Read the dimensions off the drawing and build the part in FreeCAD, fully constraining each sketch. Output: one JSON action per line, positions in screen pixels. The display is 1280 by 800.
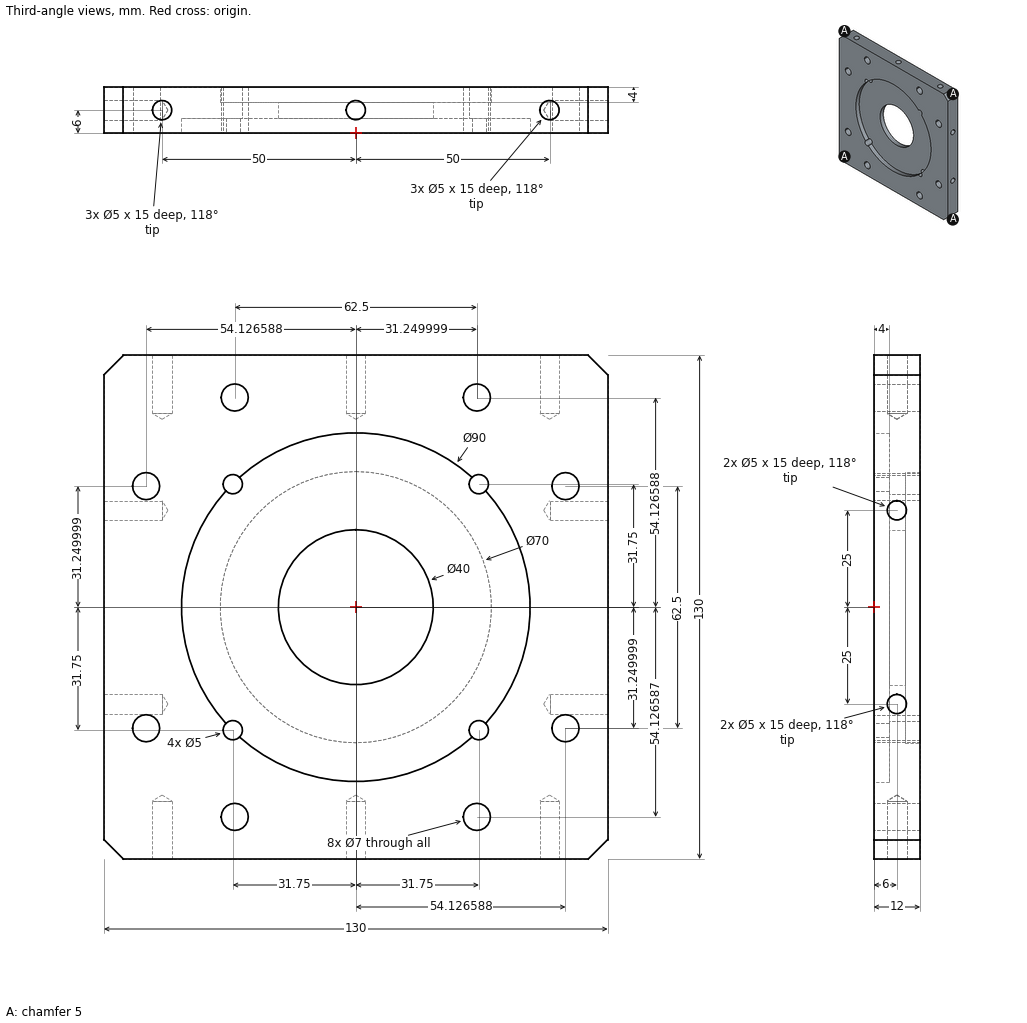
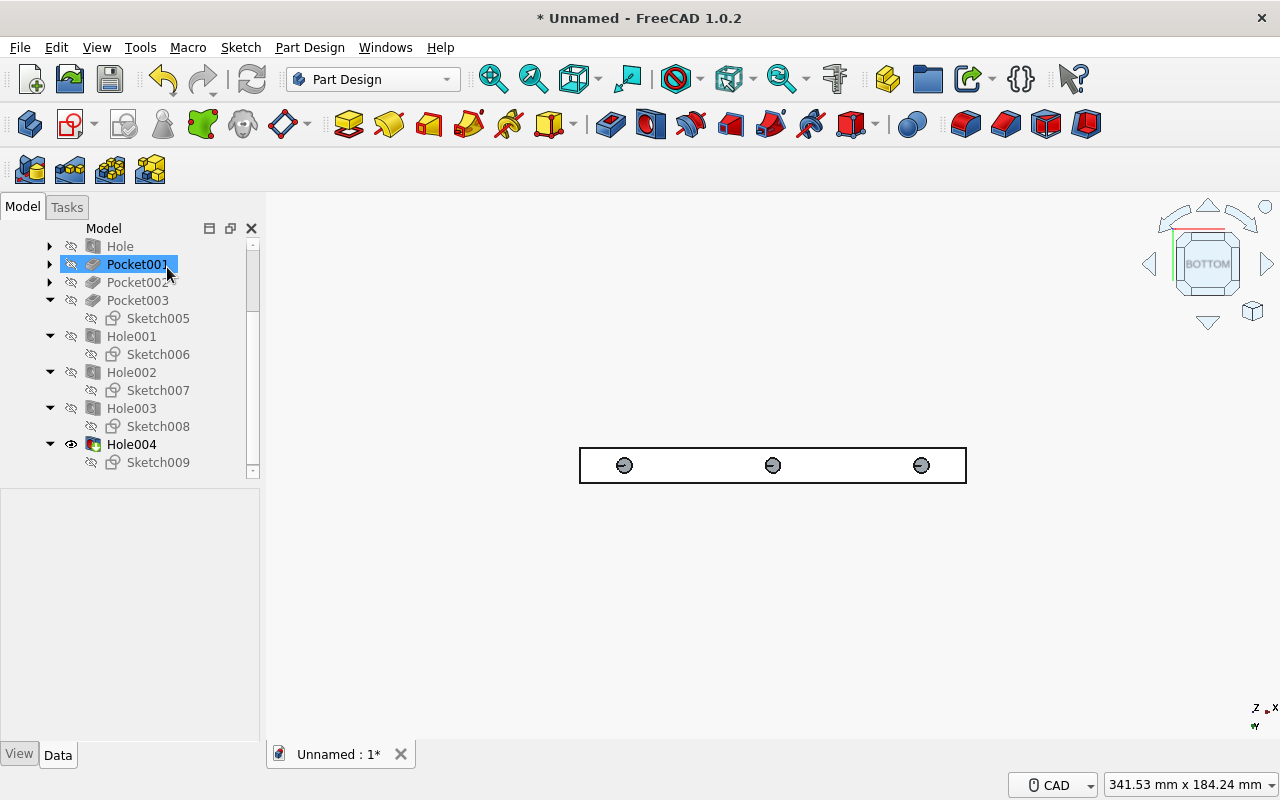
{"action": "left_click", "coordinate": [580, 464]}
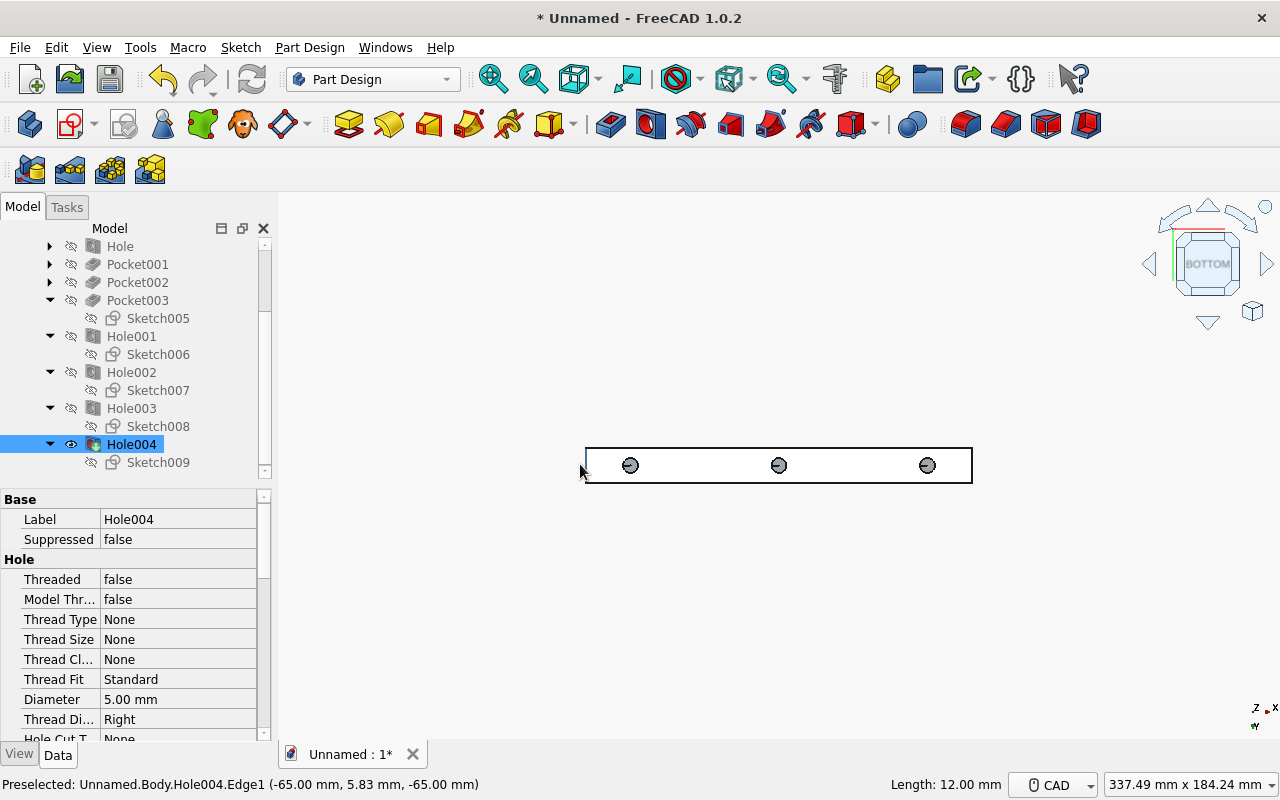
{"action": "left_click", "coordinate": [972, 464], "text": "ctrl"}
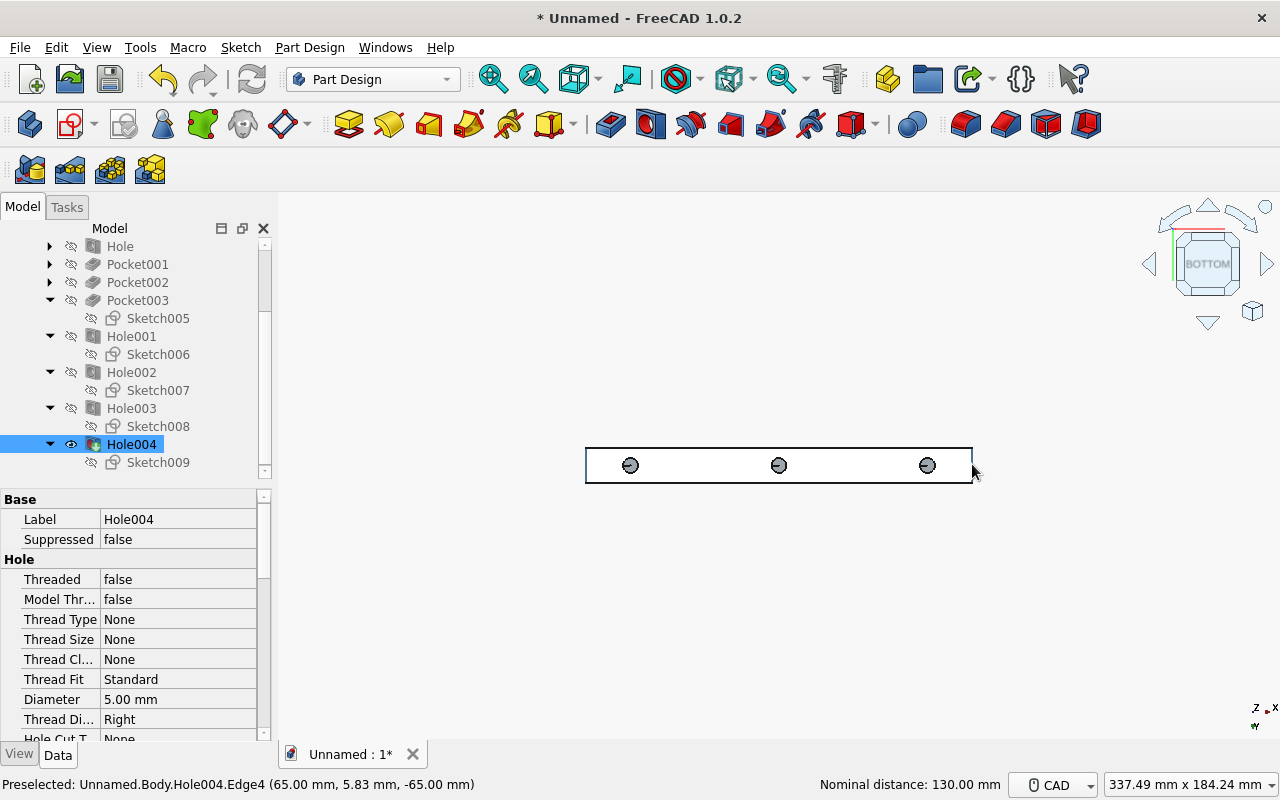
{"action": "key", "text": "0"}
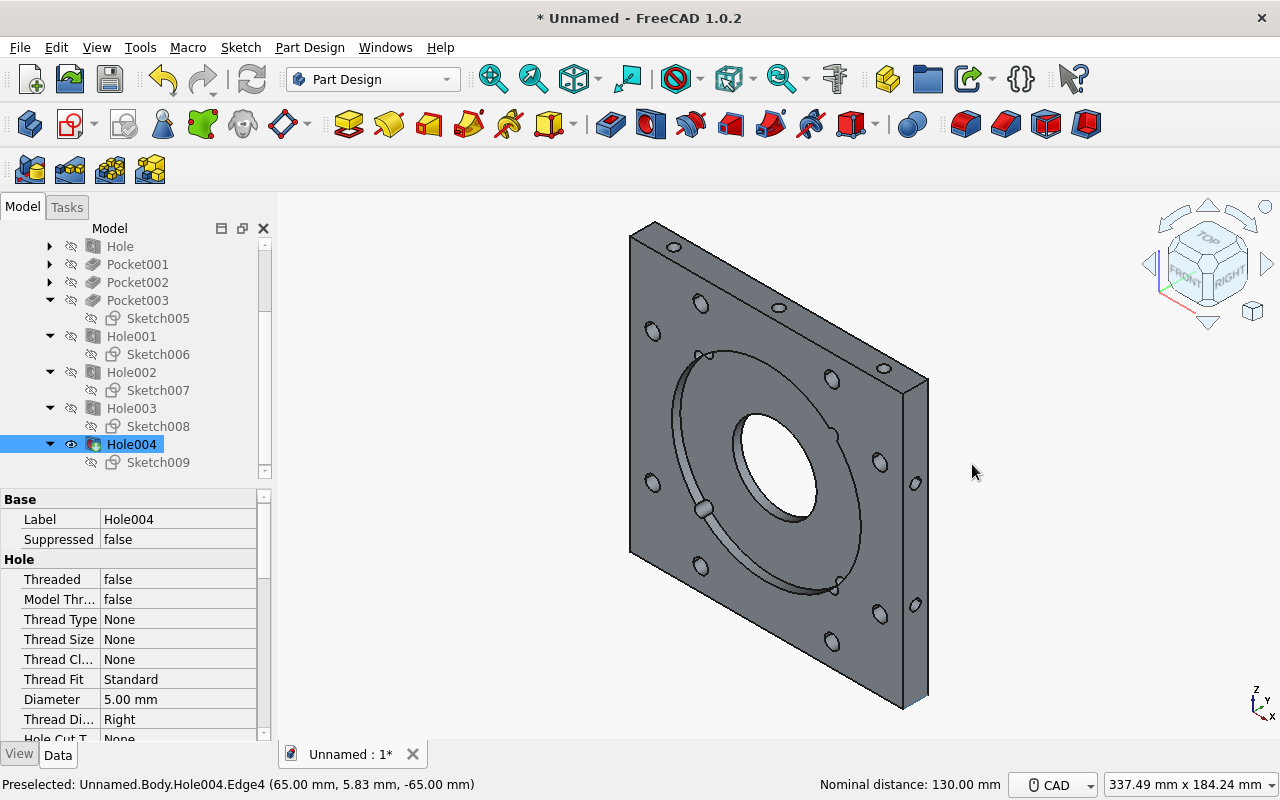
{"action": "left_click", "coordinate": [915, 386], "text": "ctrl"}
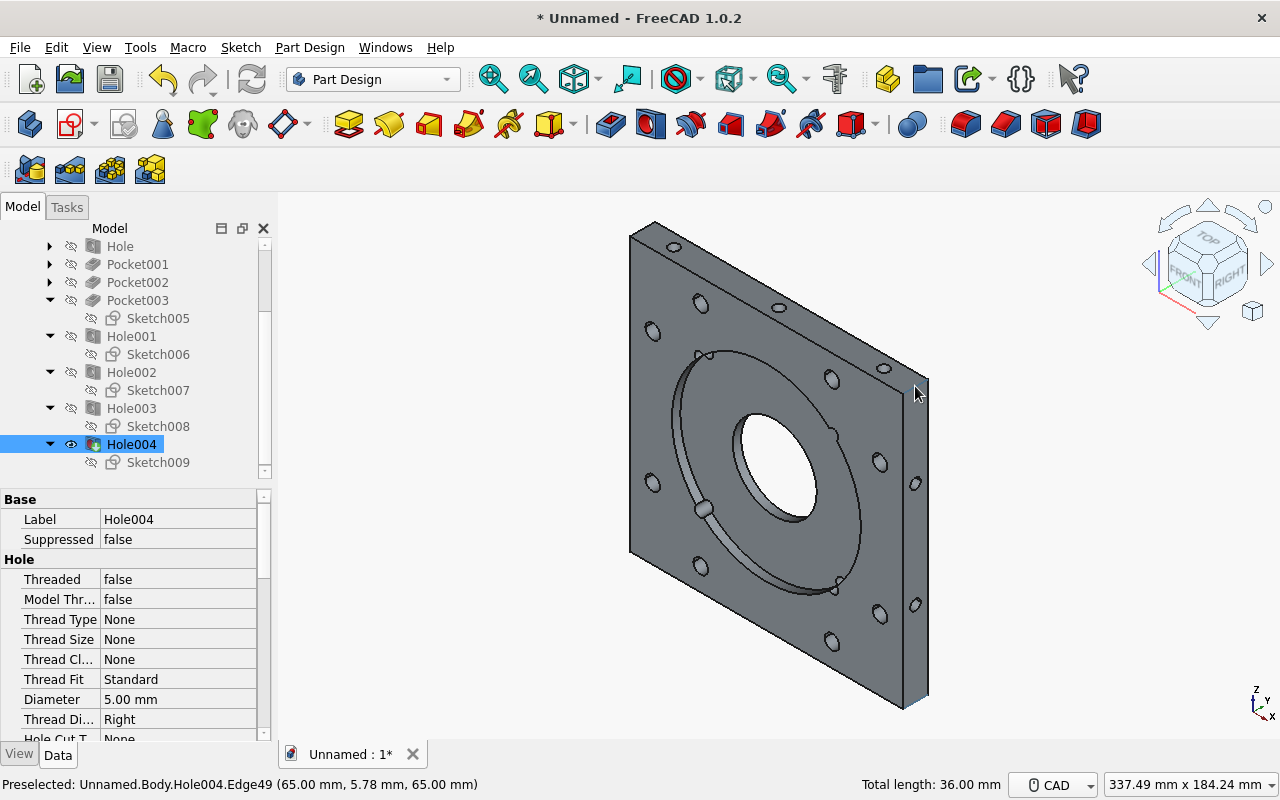
{"action": "key", "text": "2"}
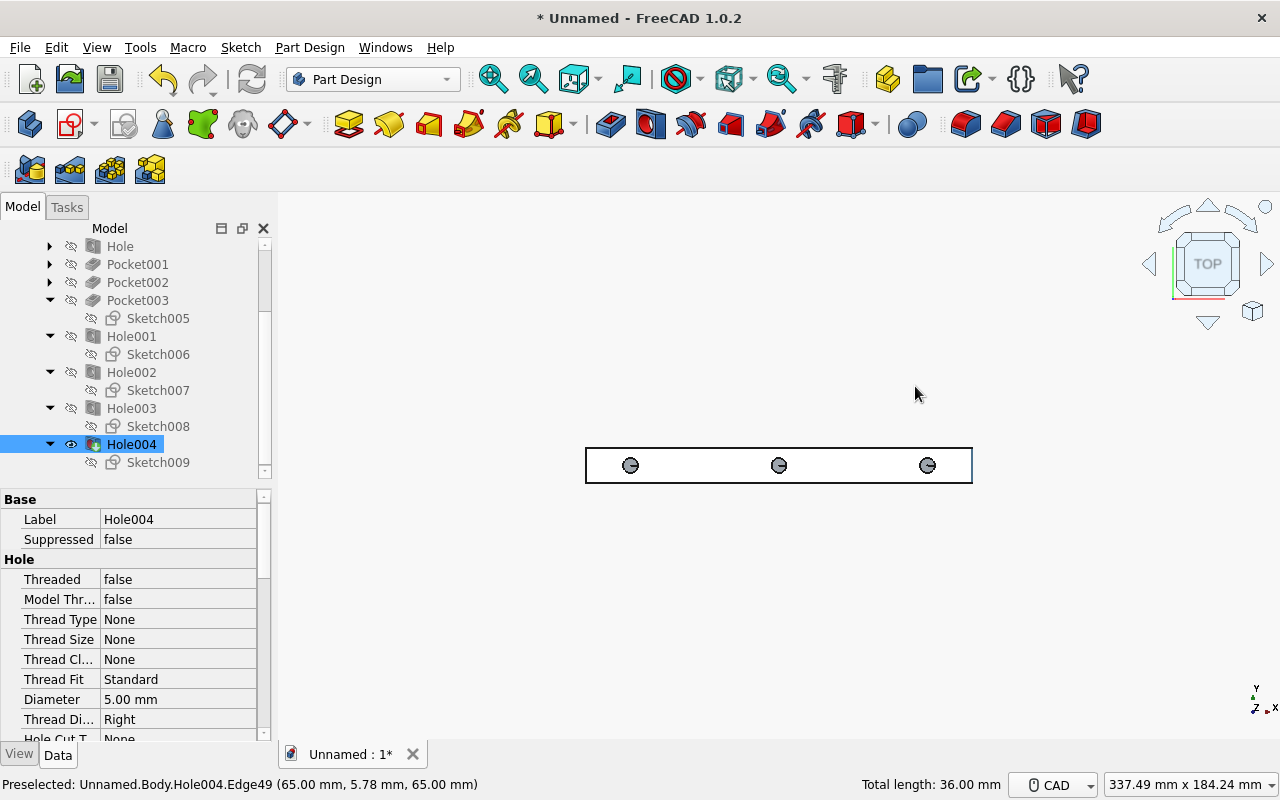
{"action": "left_click", "coordinate": [494, 80]}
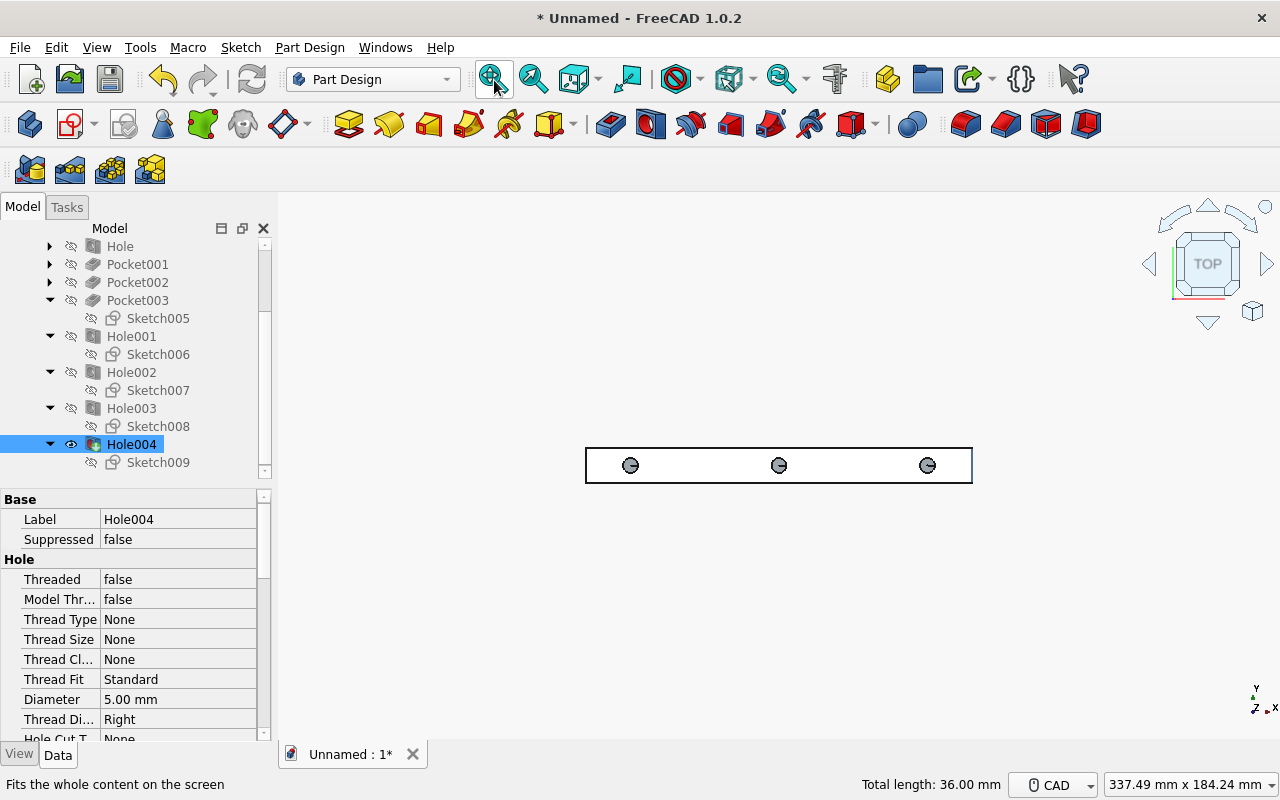
{"action": "left_click", "coordinate": [586, 464], "text": "ctrl"}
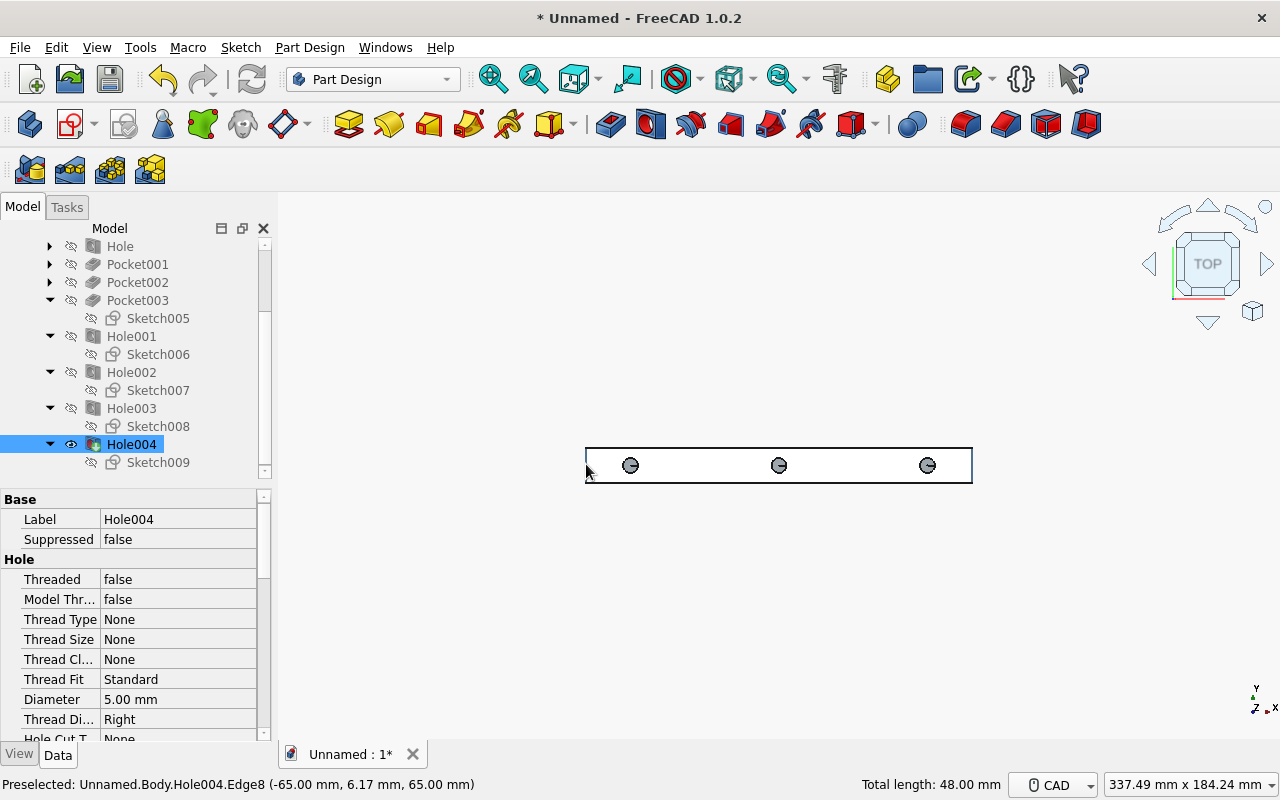
{"action": "left_click", "coordinate": [1006, 124]}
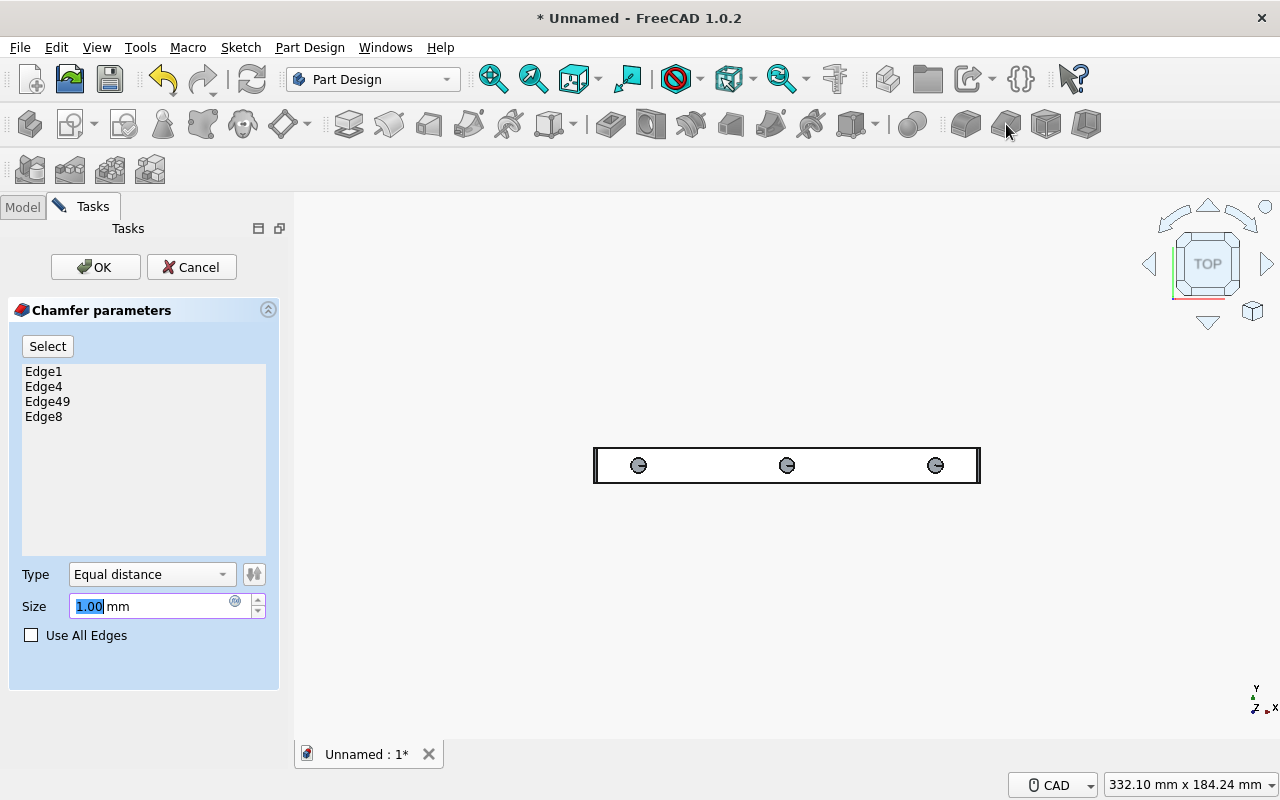
{"action": "type", "text": "5"}
{"action": "key", "text": "Tab"}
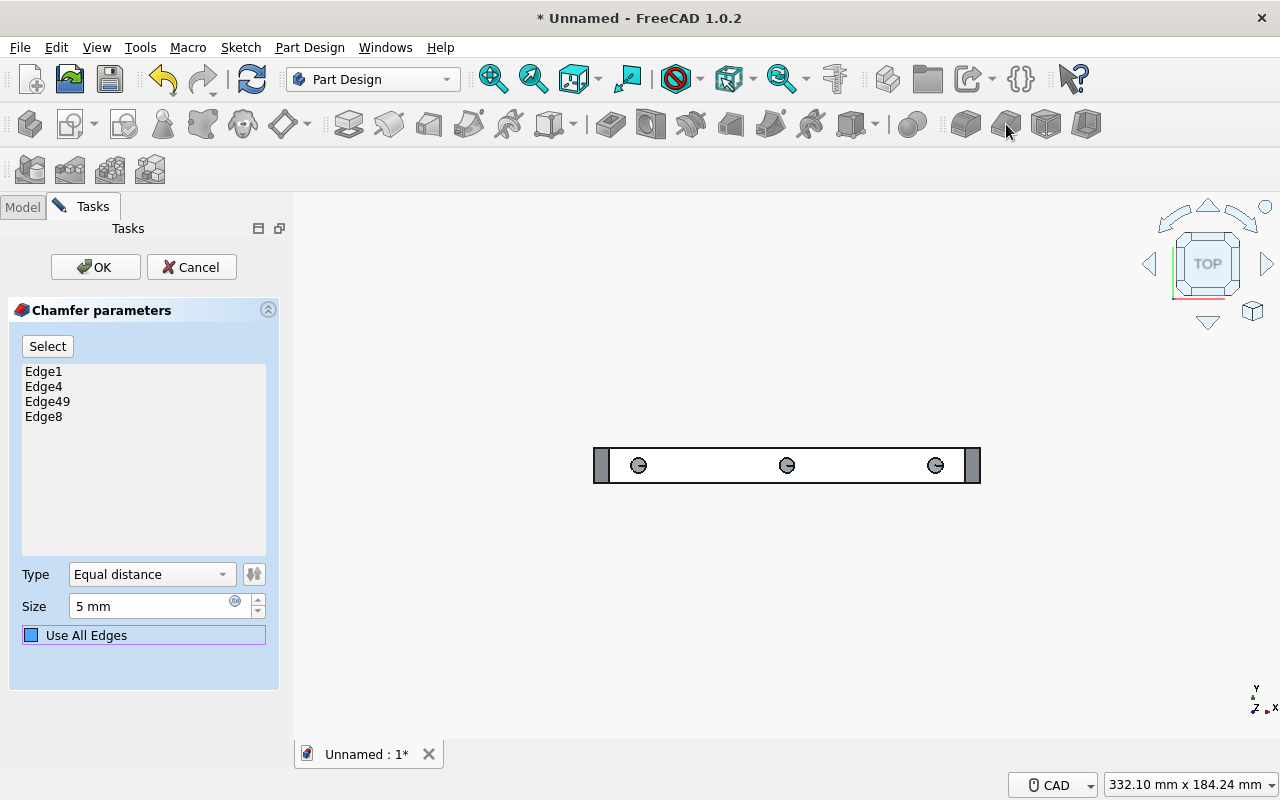
{"action": "left_click", "coordinate": [96, 267]}